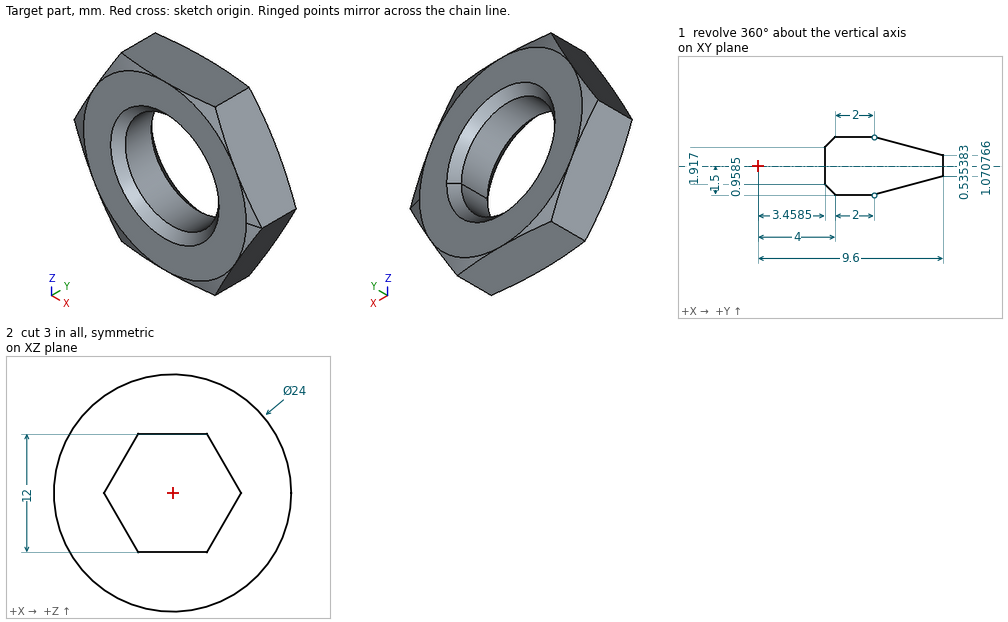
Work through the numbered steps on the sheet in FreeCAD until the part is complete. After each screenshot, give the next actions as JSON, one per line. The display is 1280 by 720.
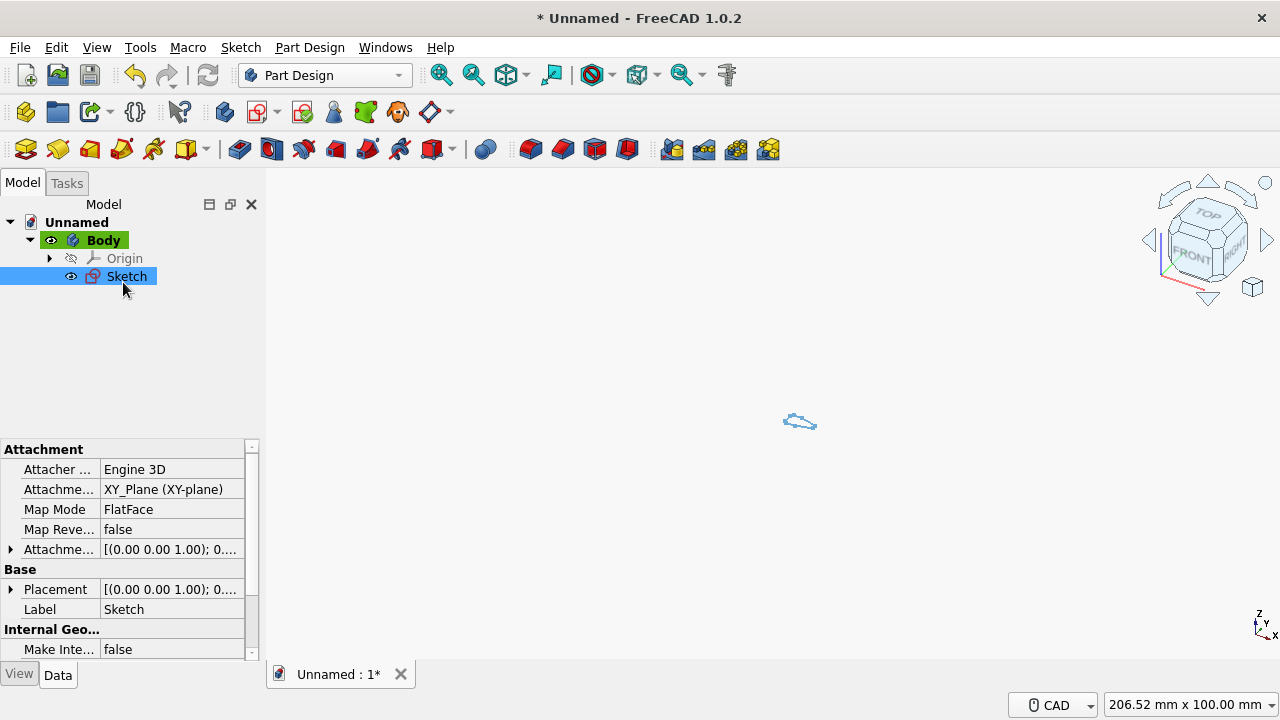
{"action": "left_click", "coordinate": [58, 150]}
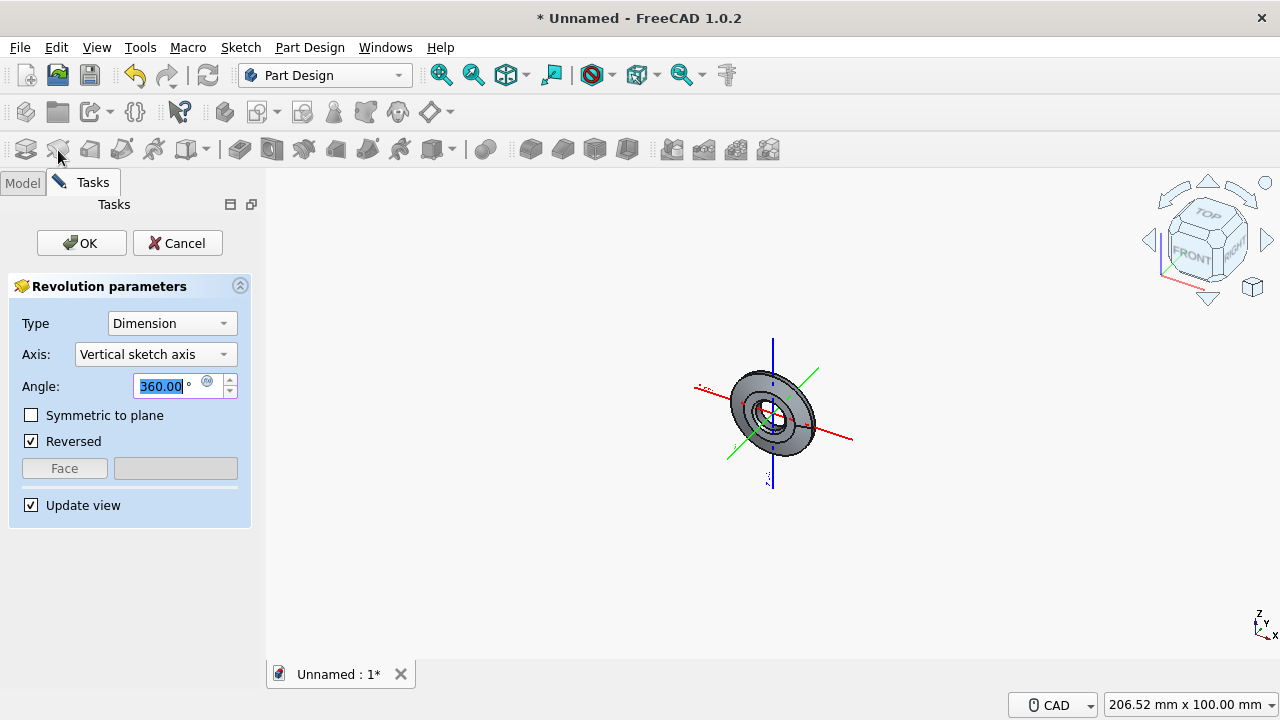
{"action": "left_click", "coordinate": [82, 243]}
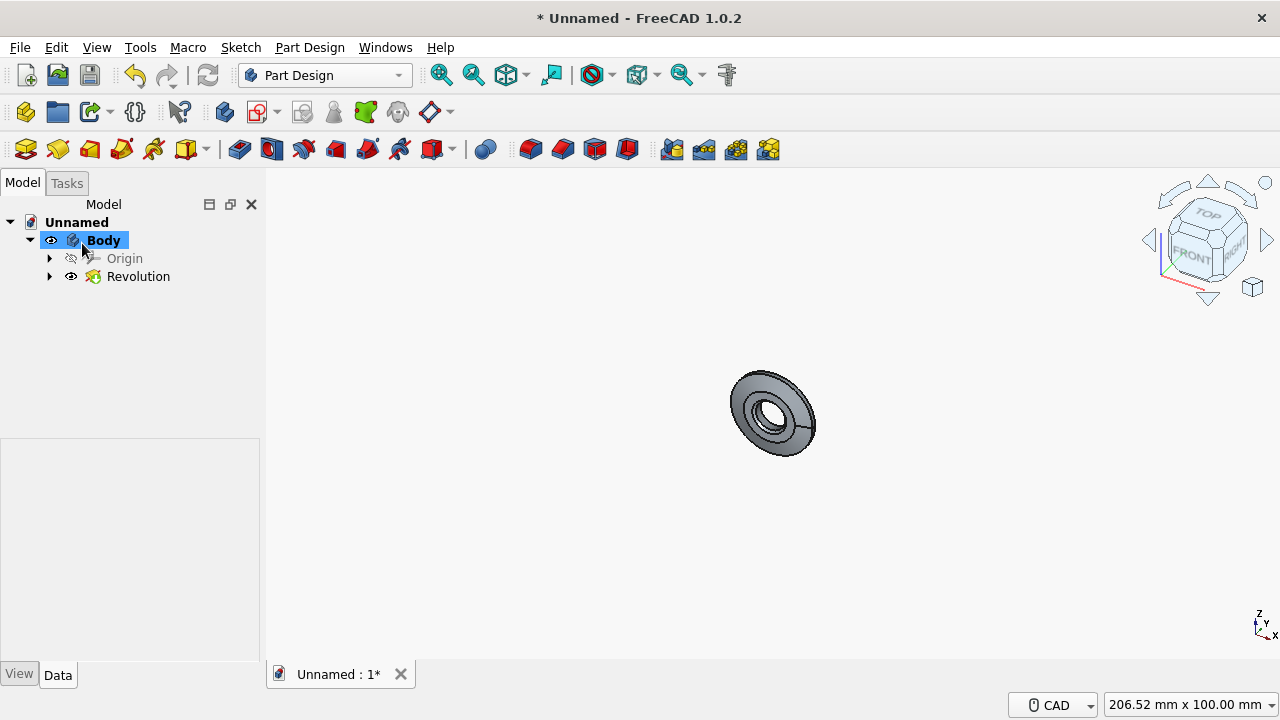
{"action": "left_click", "coordinate": [442, 76]}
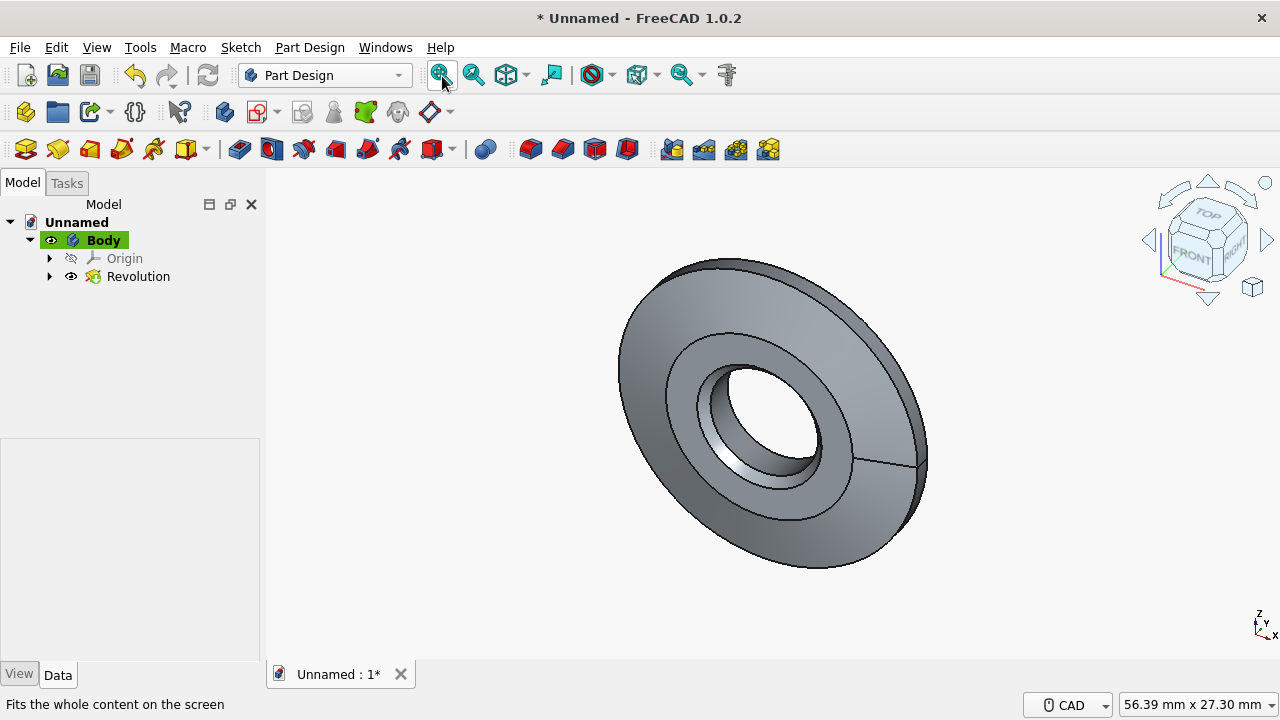
{"action": "left_click", "coordinate": [258, 112]}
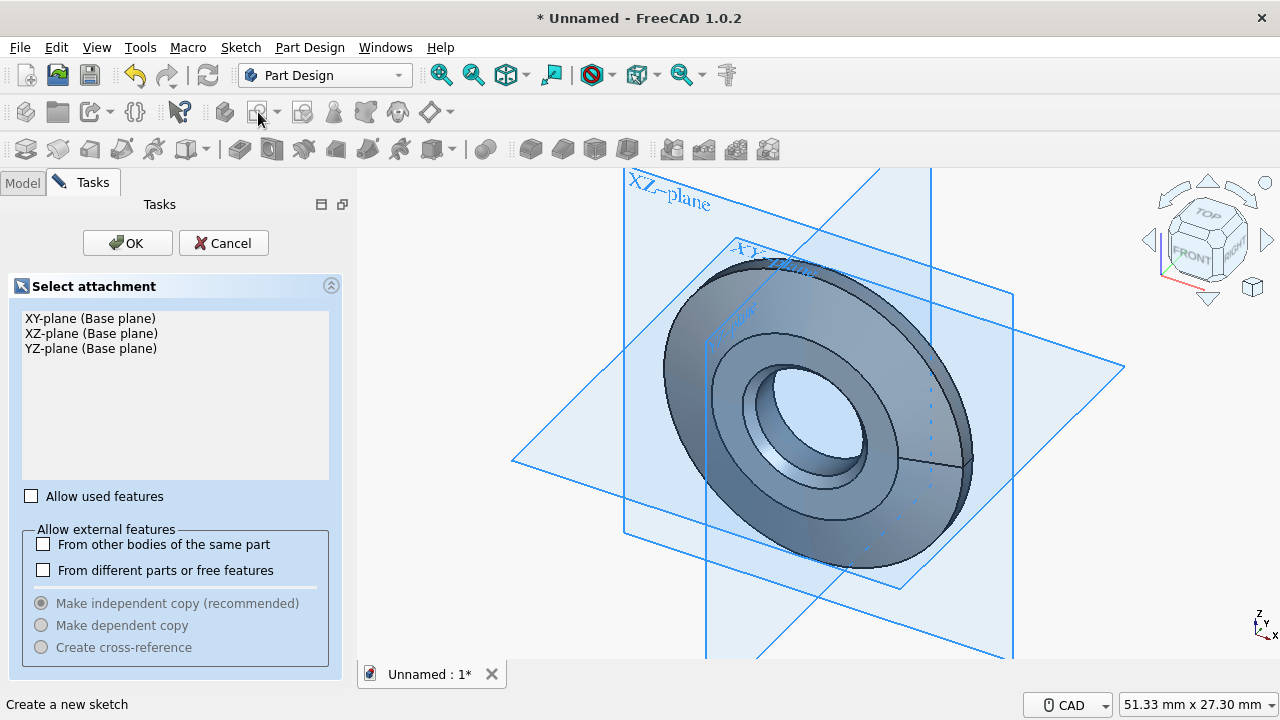
{"action": "left_click", "coordinate": [82, 334]}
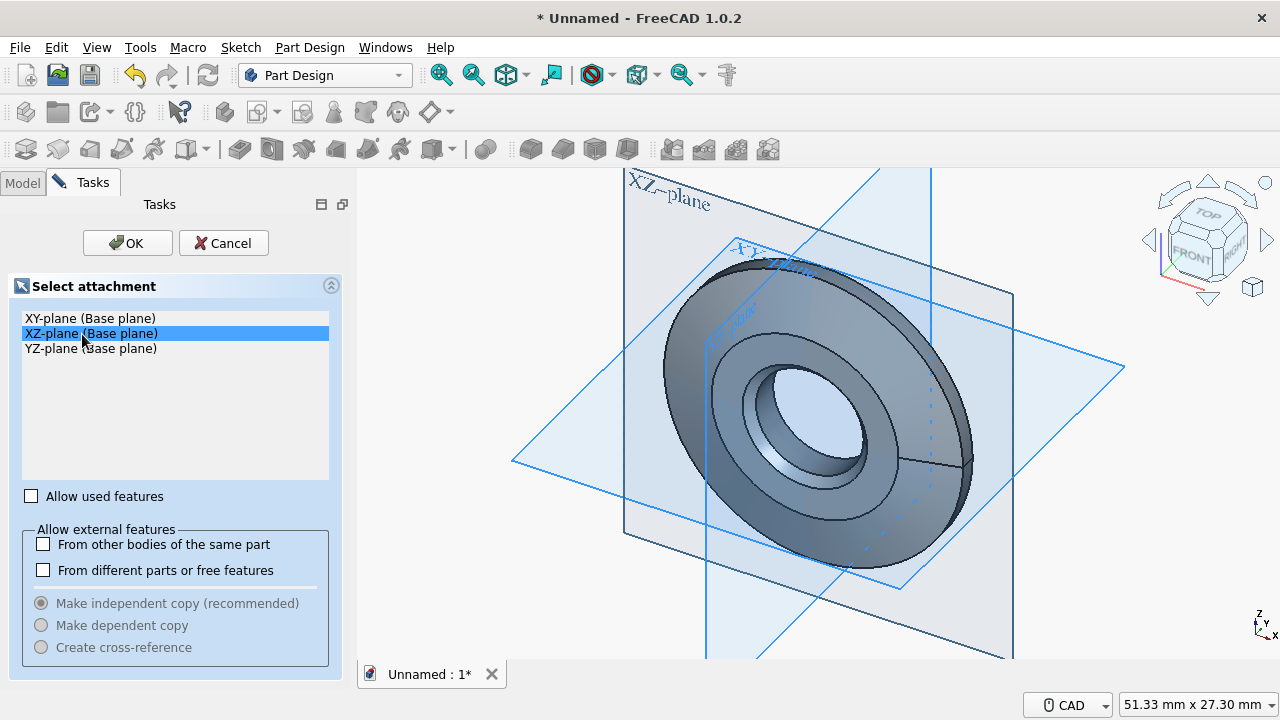
{"action": "left_click", "coordinate": [128, 243]}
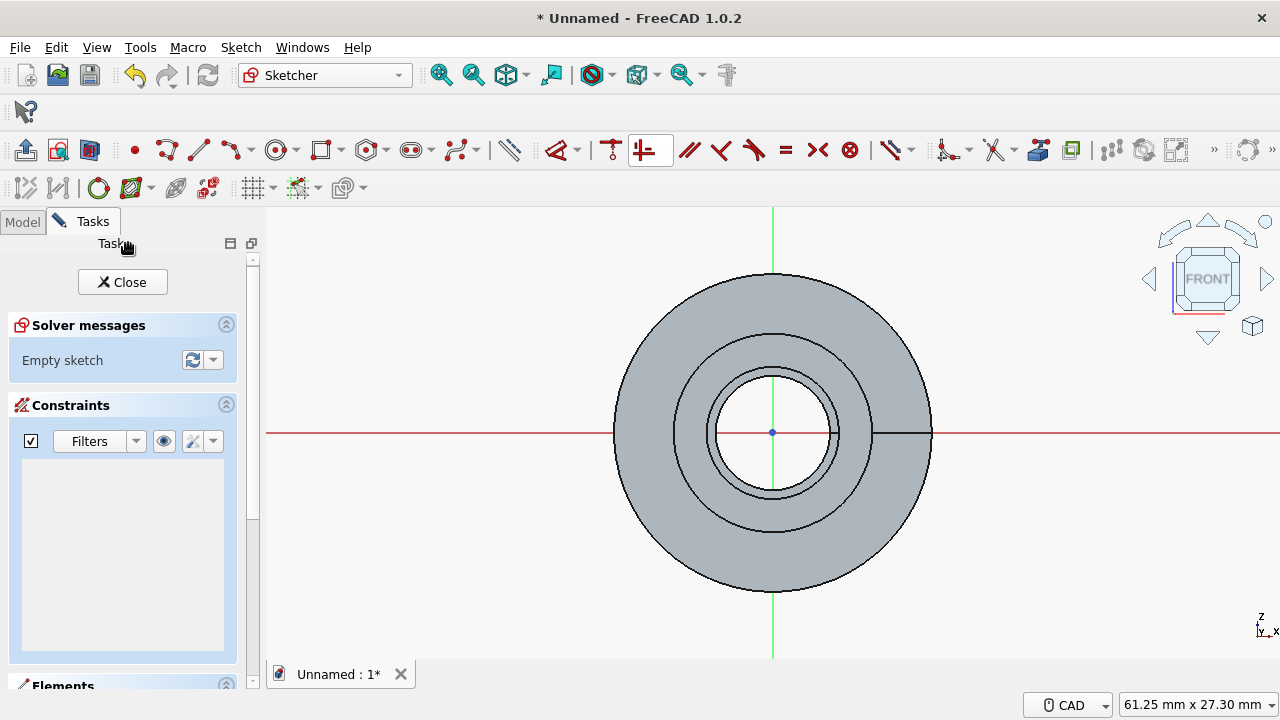
{"action": "left_click", "coordinate": [90, 150]}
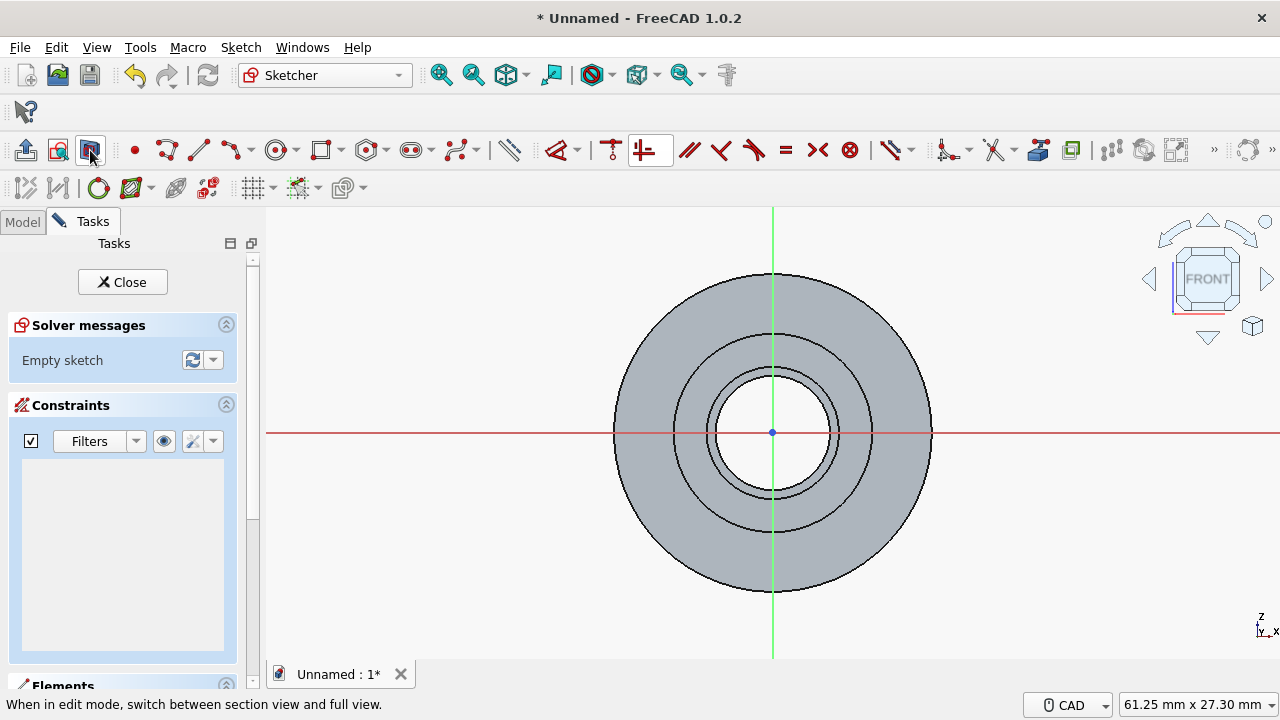
{"action": "scroll", "coordinate": [565, 433], "scroll_direction": "down", "scroll_amount": 2}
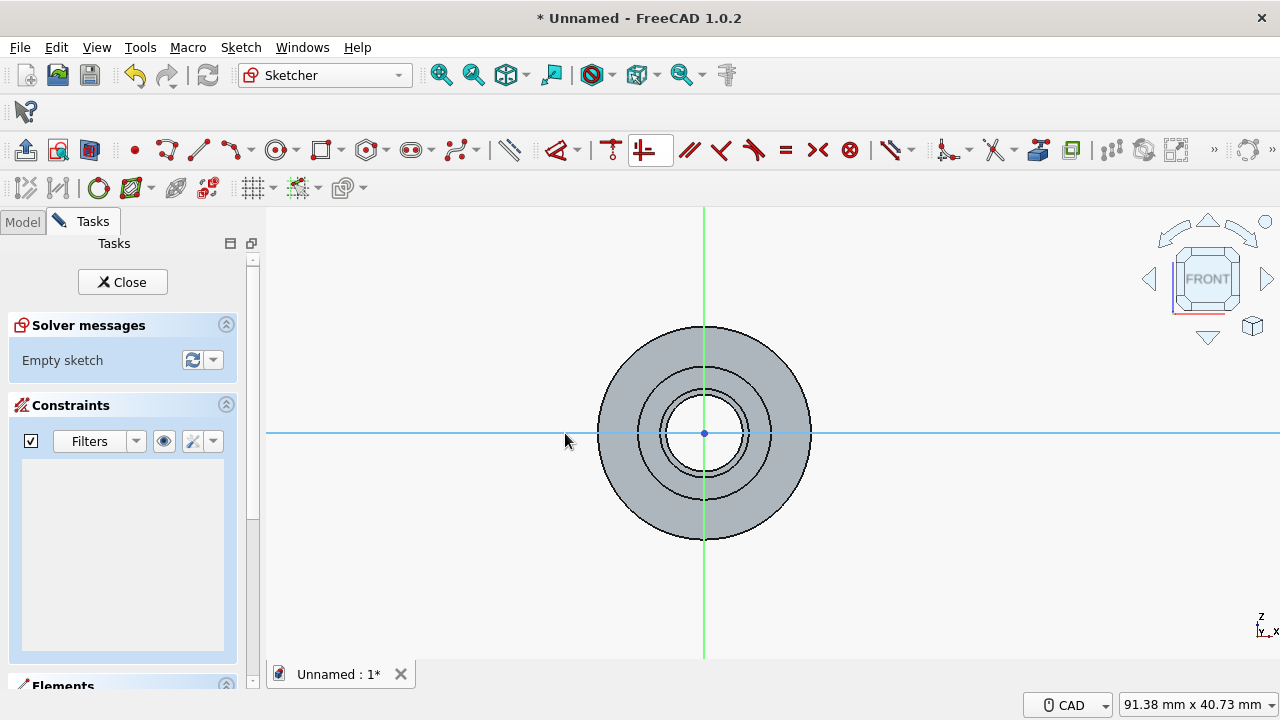
{"action": "left_click", "coordinate": [366, 150]}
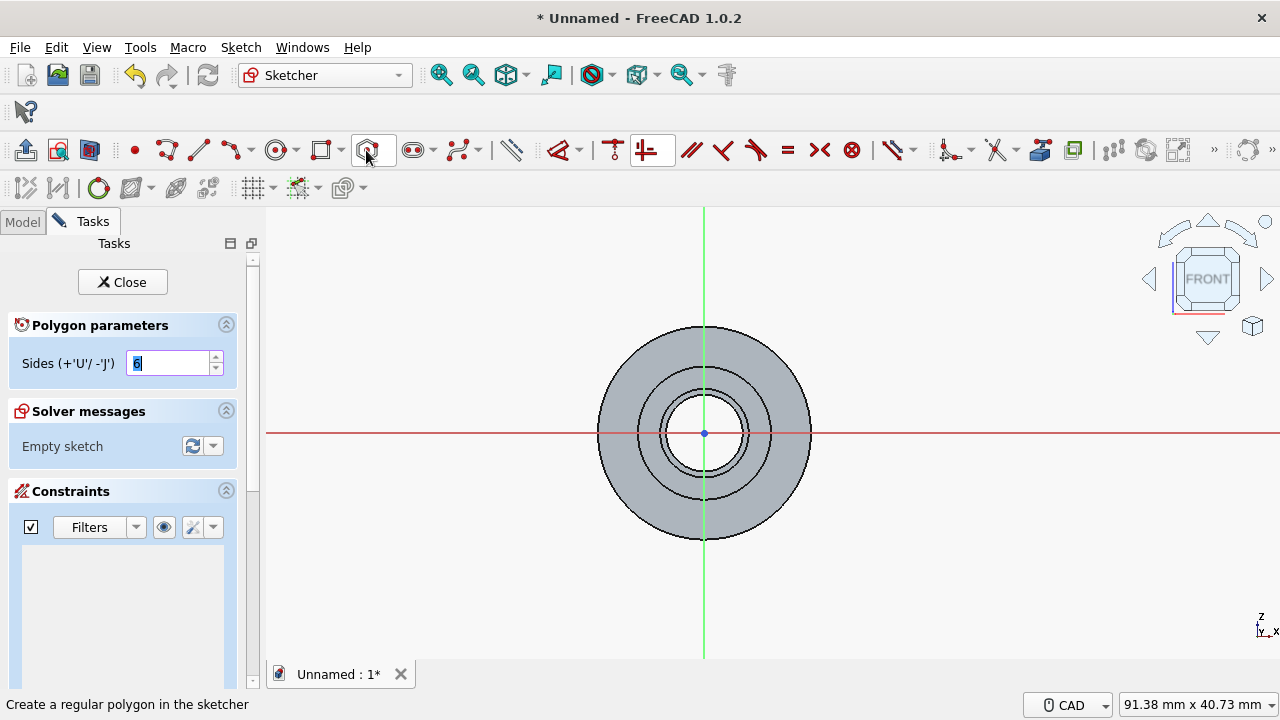
{"action": "left_click", "coordinate": [704, 433]}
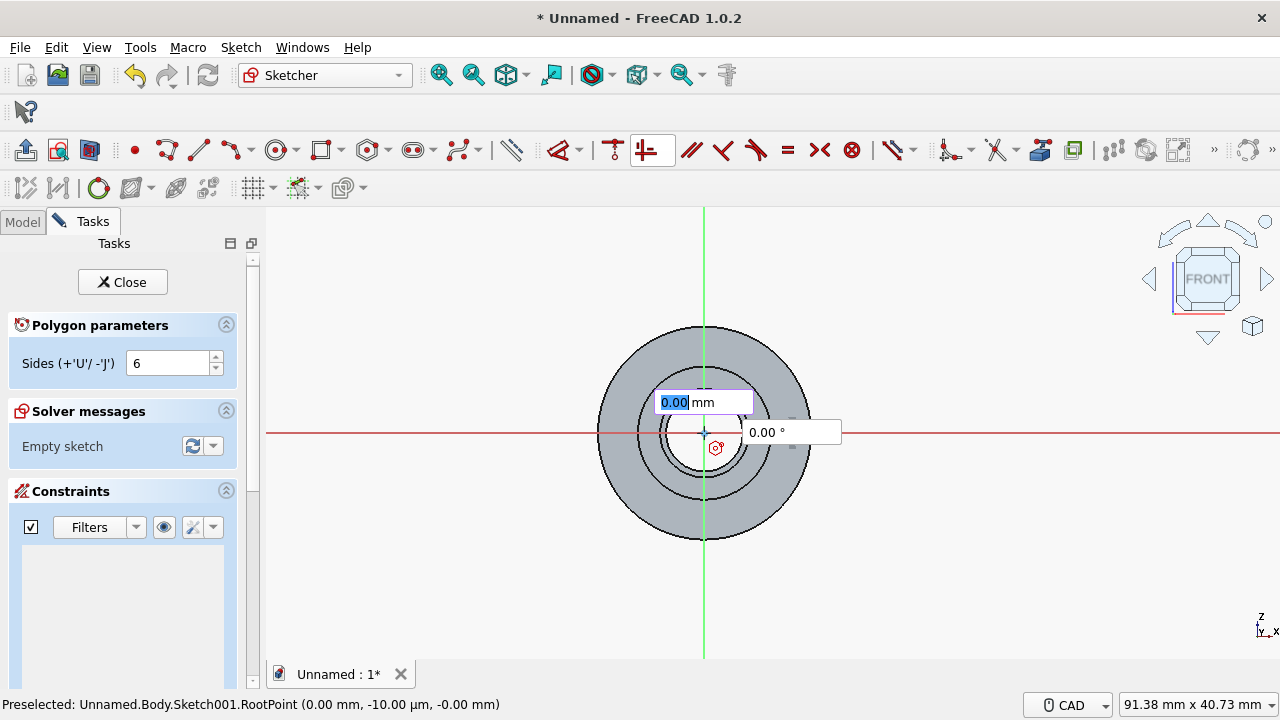
{"action": "left_click", "coordinate": [628, 433]}
{"action": "key", "text": "Escape"}